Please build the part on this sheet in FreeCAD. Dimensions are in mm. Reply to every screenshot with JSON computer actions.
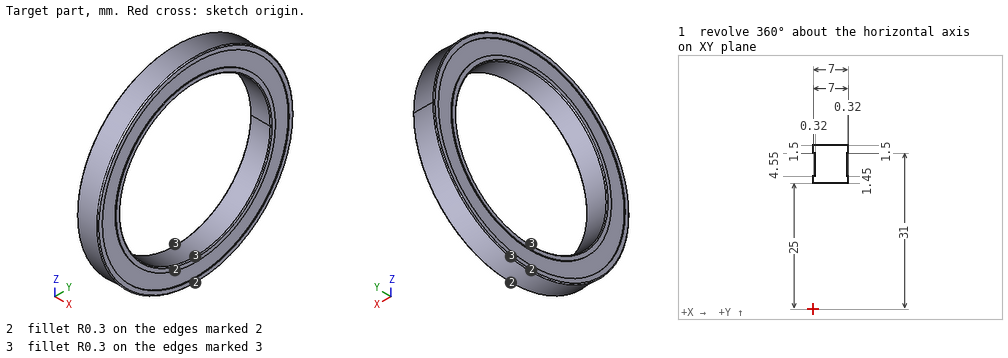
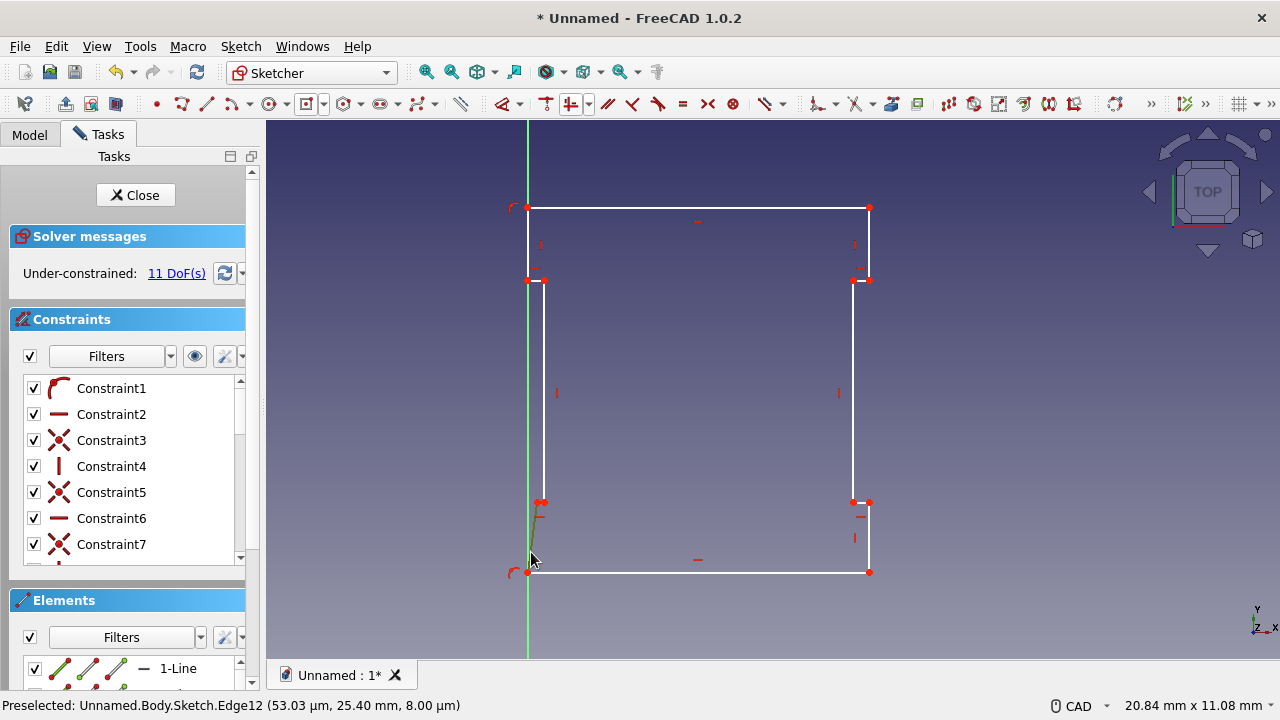
{"action": "key", "text": "v"}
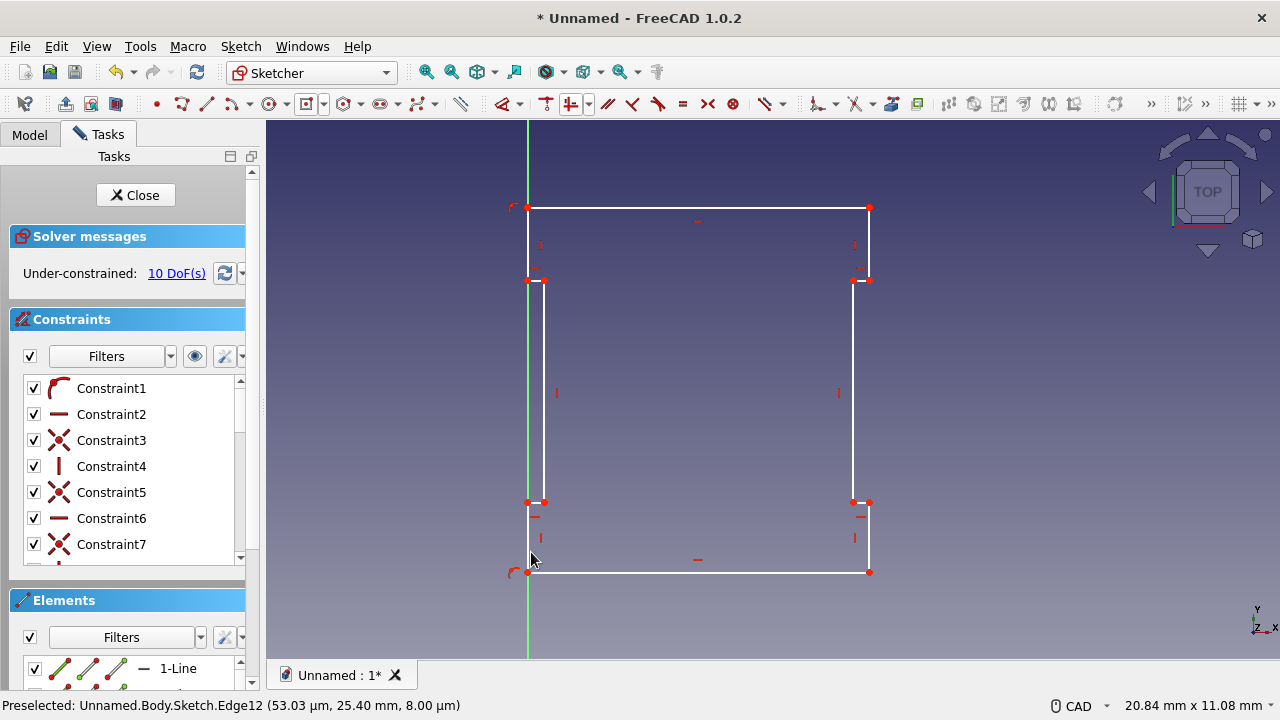
{"action": "left_click", "coordinate": [630, 573]}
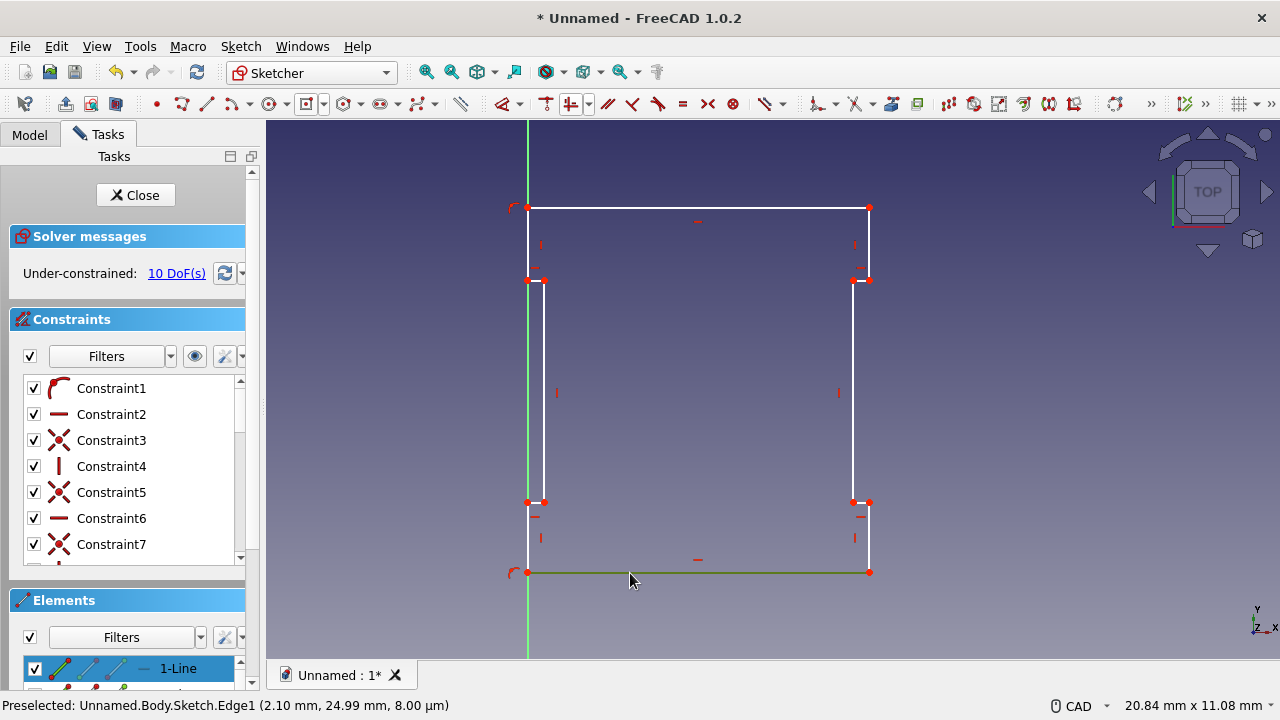
{"action": "left_click", "coordinate": [520, 104]}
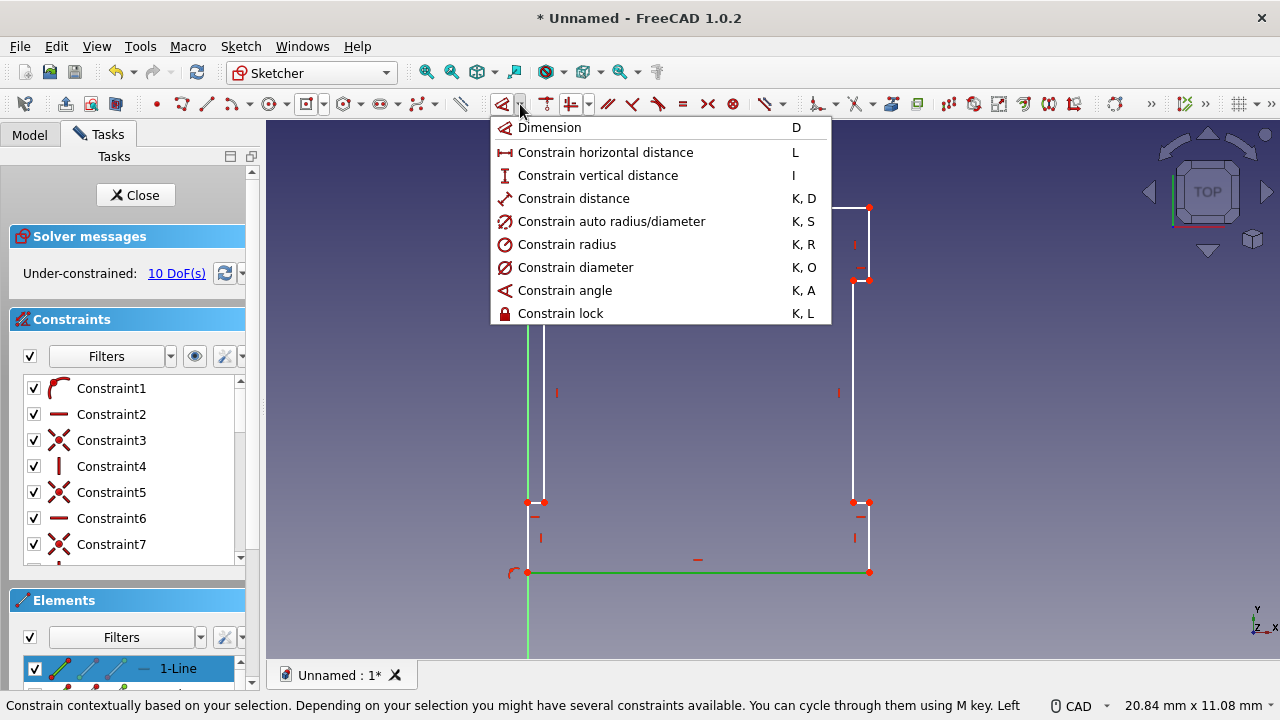
{"action": "left_click", "coordinate": [661, 152]}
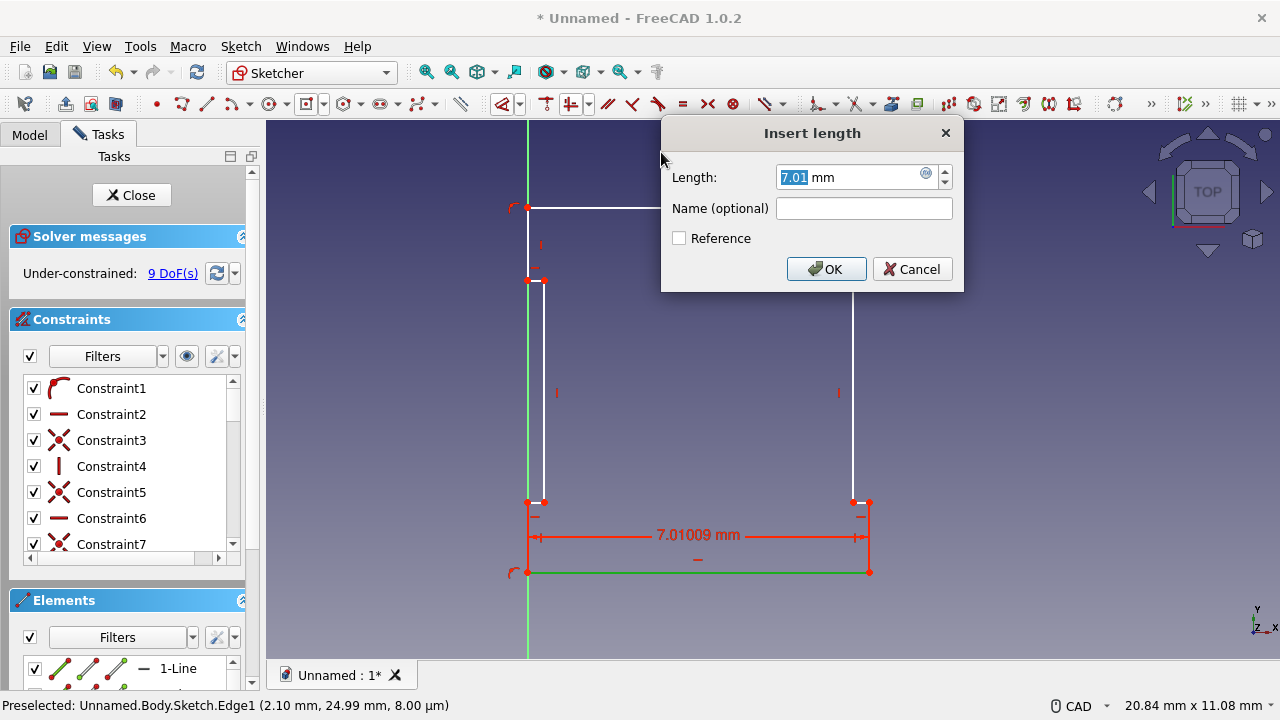
{"action": "type", "text": "7"}
{"action": "key", "text": "Return"}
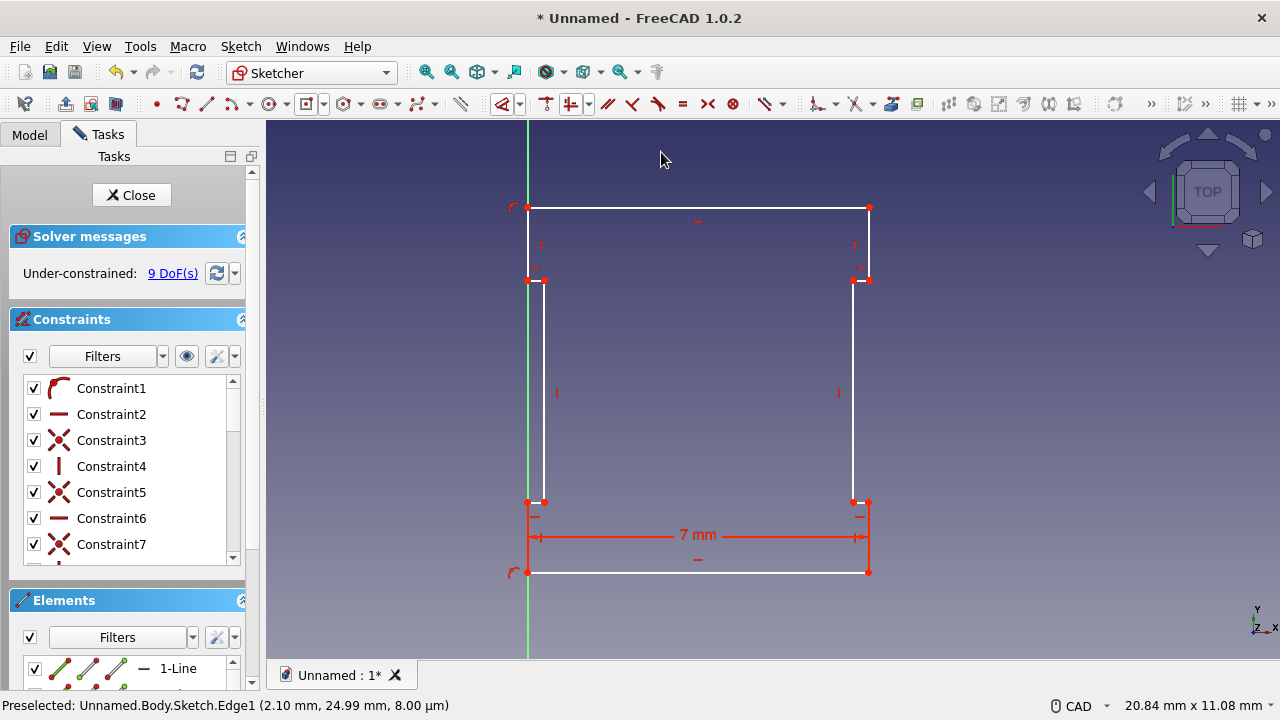
{"action": "left_click", "coordinate": [767, 208]}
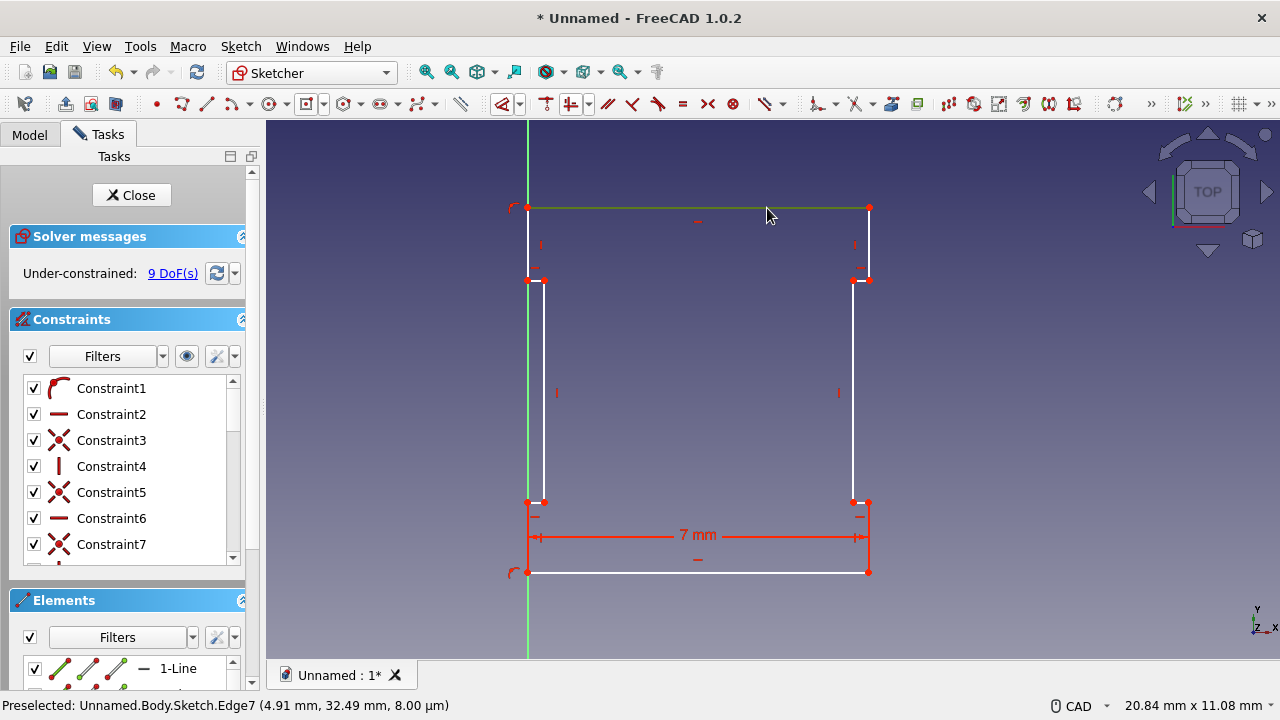
{"action": "left_click", "coordinate": [520, 104]}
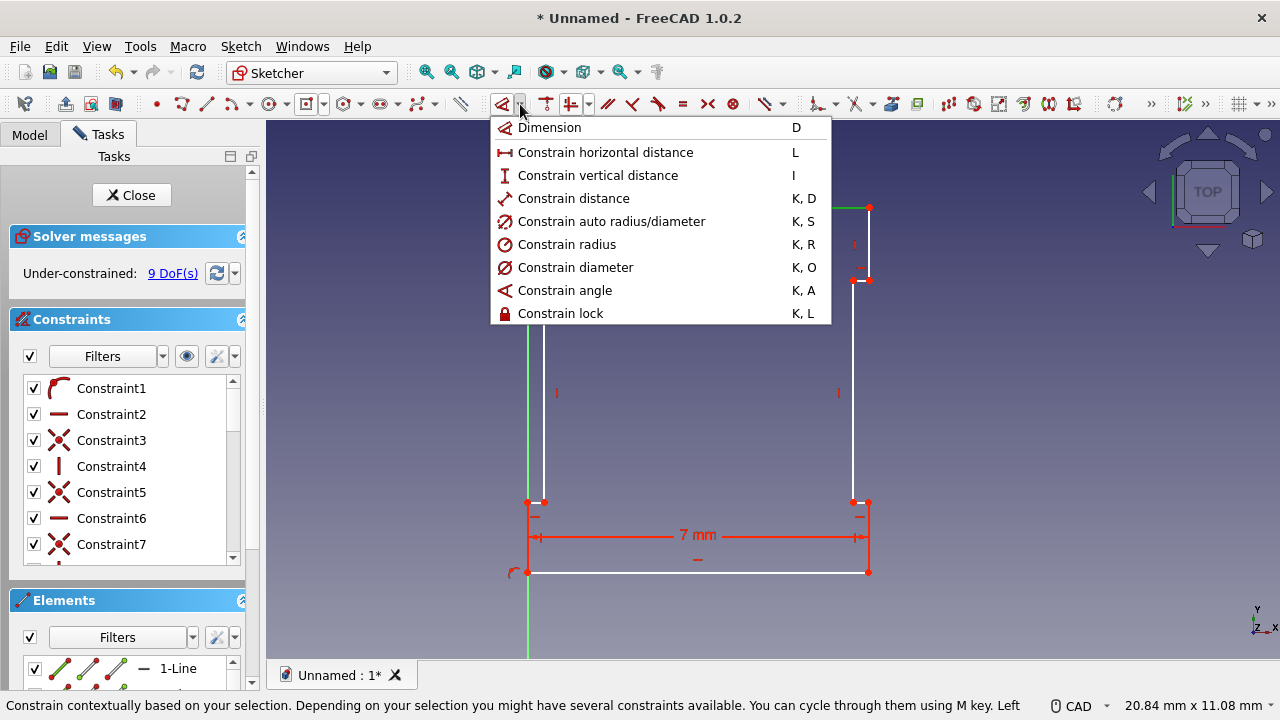
{"action": "left_click", "coordinate": [661, 152]}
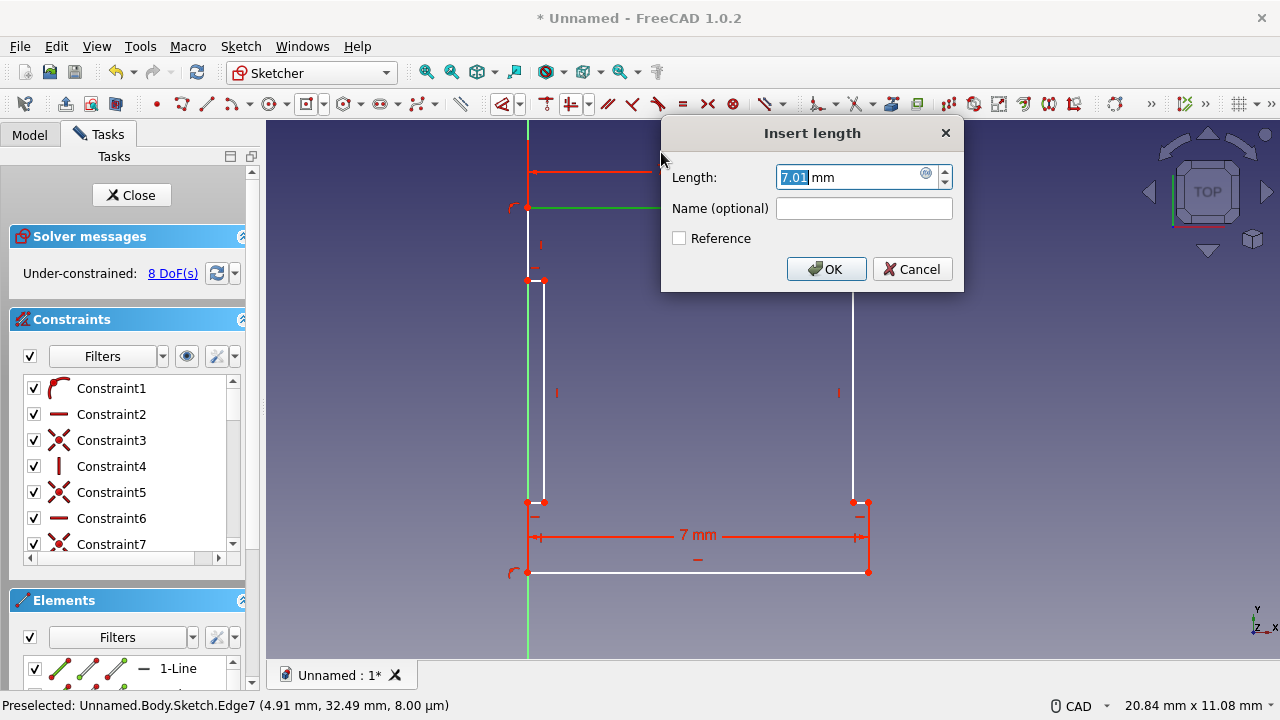
{"action": "type", "text": "7"}
{"action": "key", "text": "Return"}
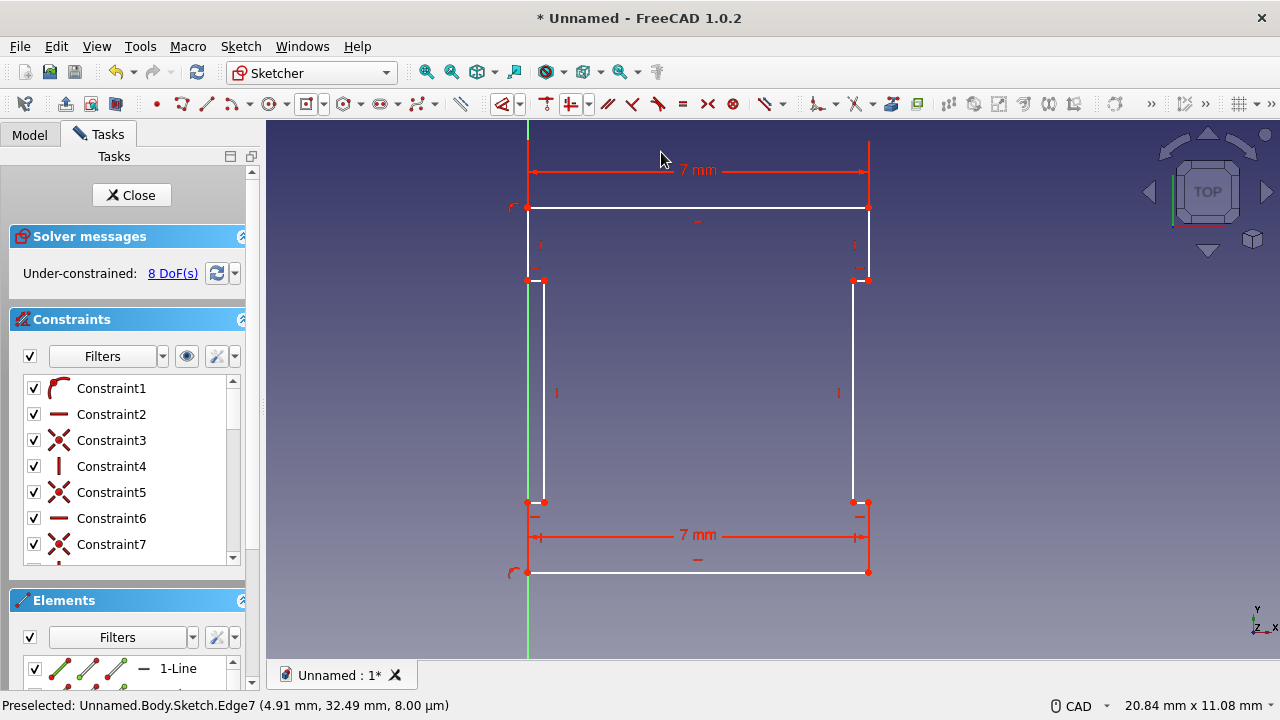
{"action": "left_click", "coordinate": [869, 259]}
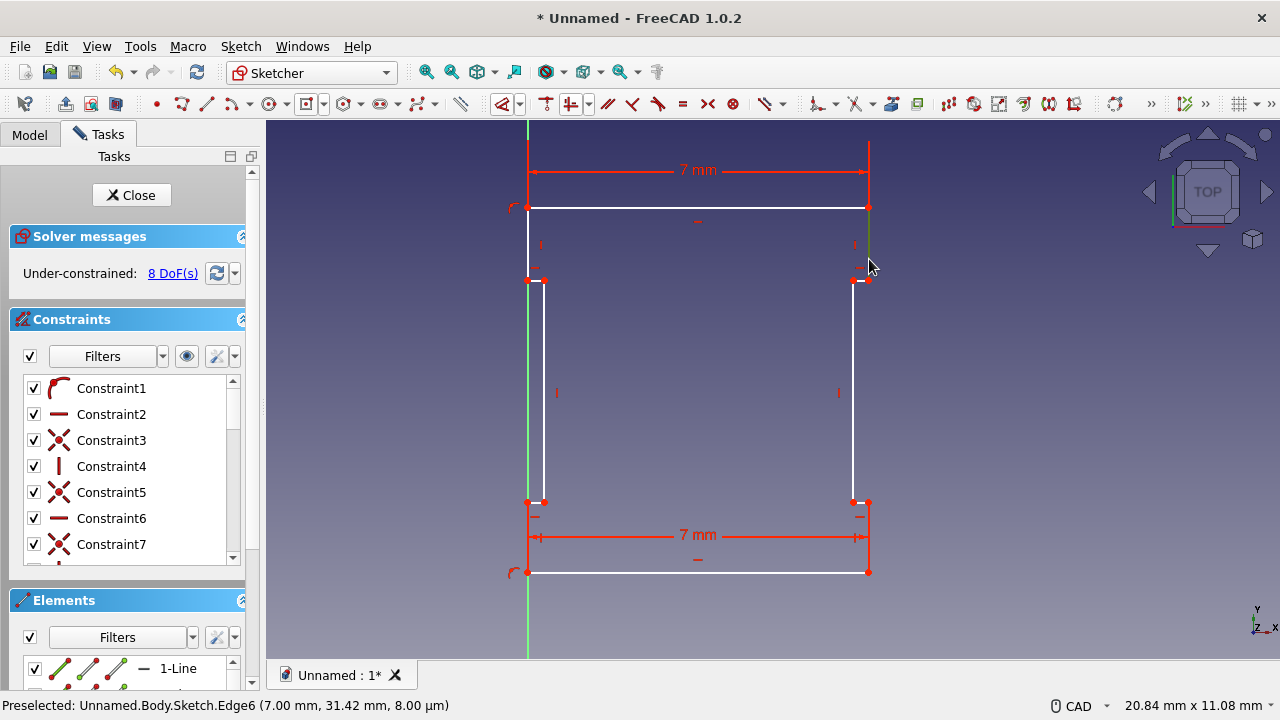
{"action": "key", "text": "i"}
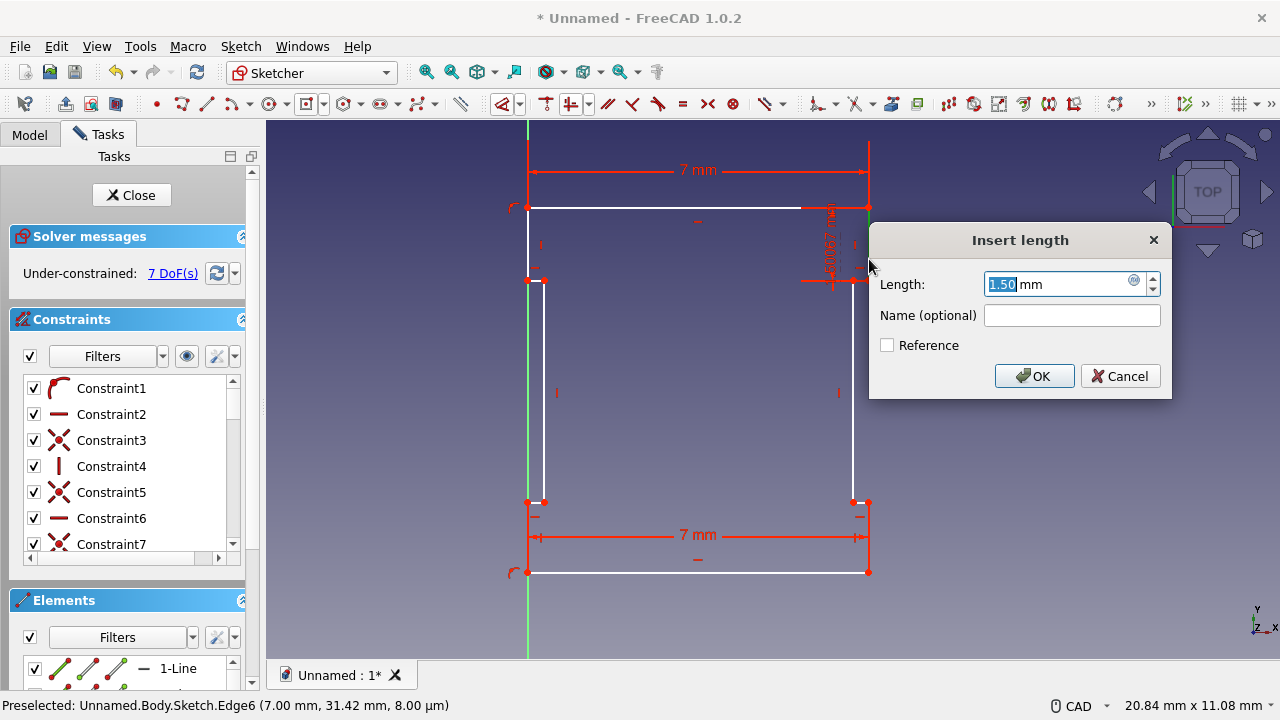
{"action": "type", "text": "1.5"}
{"action": "key", "text": "Return"}